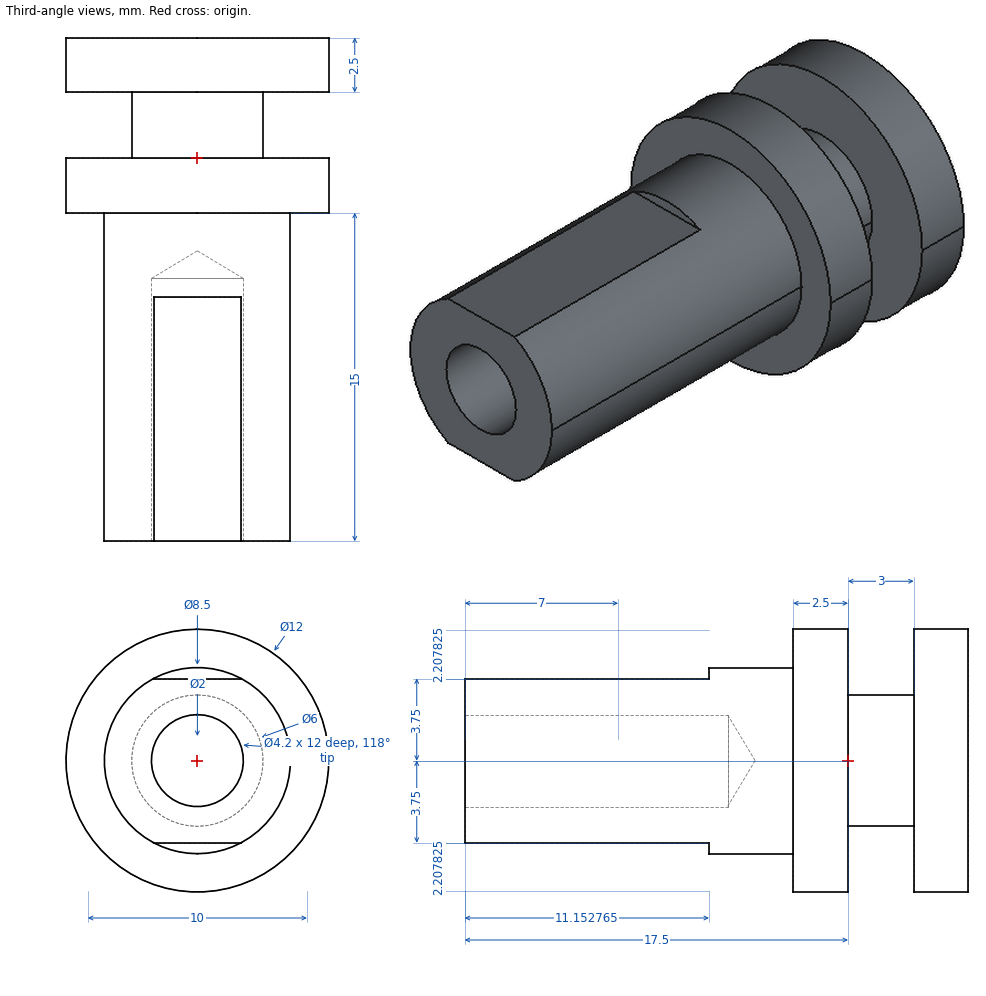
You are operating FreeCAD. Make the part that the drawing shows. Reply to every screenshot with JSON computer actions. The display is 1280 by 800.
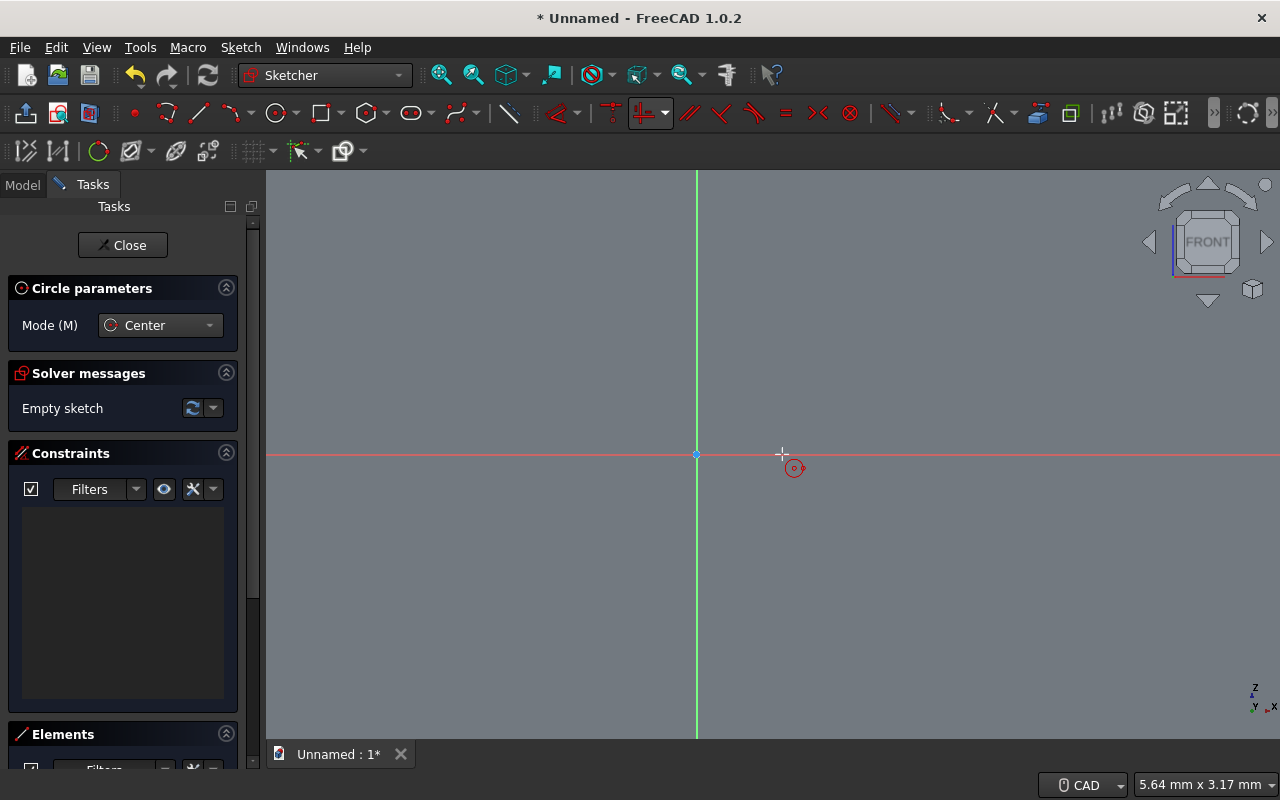
{"action": "left_click", "coordinate": [697, 454]}
{"action": "mouse_move", "coordinate": [824, 327]}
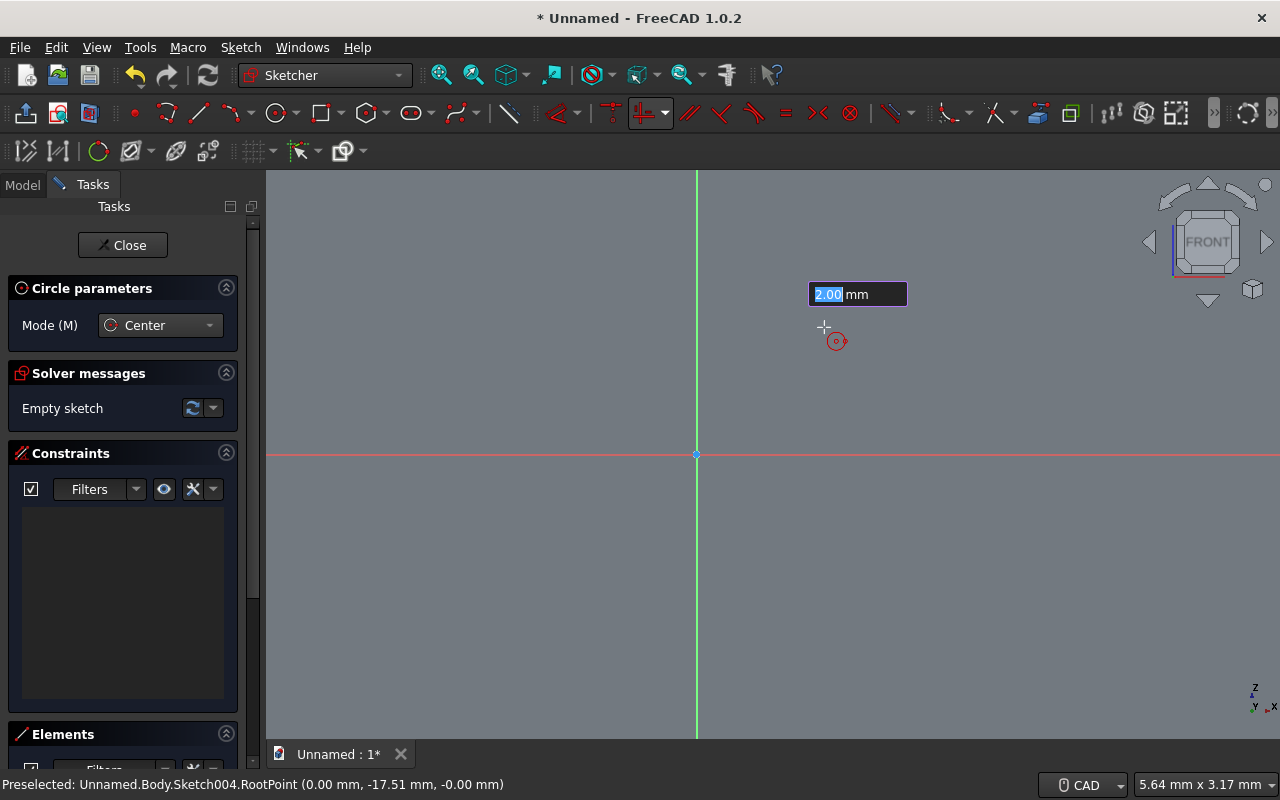
{"action": "type", "text": "2"}
{"action": "key", "text": "Return"}
{"action": "key", "text": "Escape"}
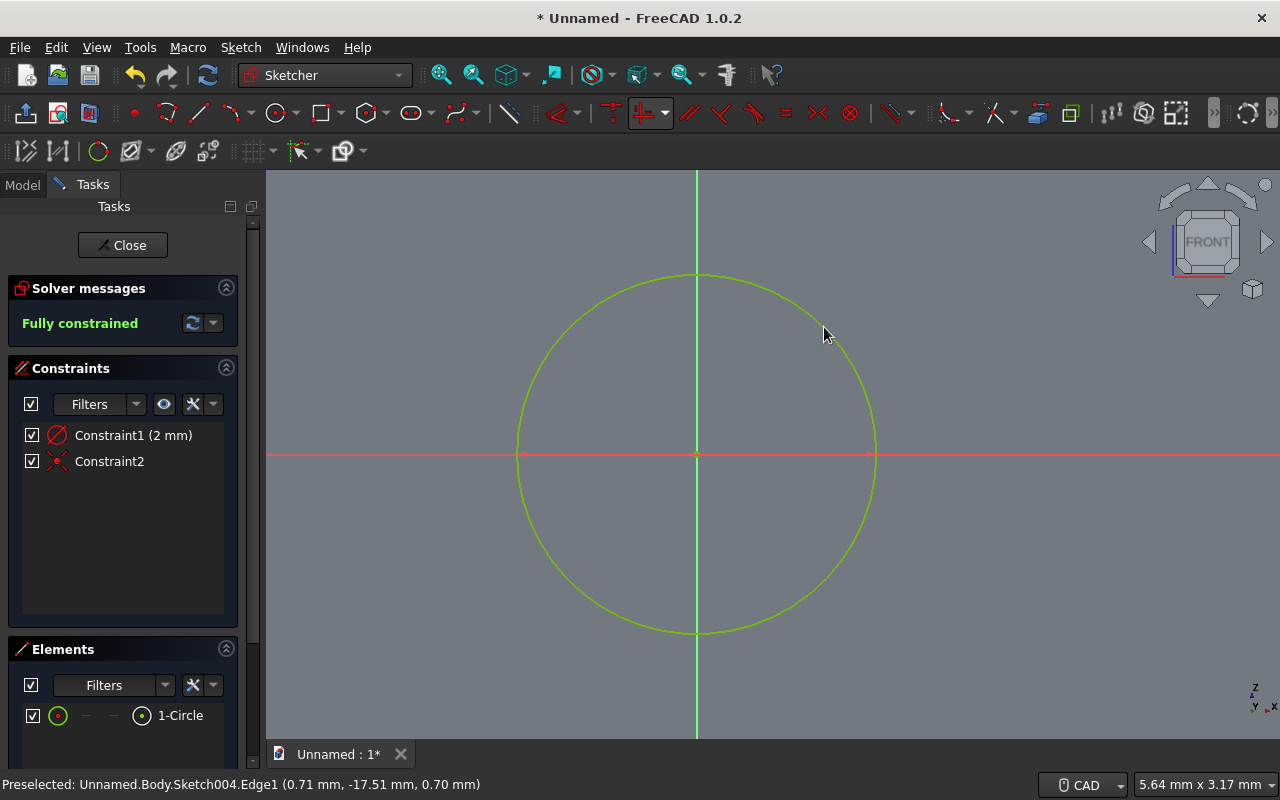
{"action": "left_click", "coordinate": [123, 245]}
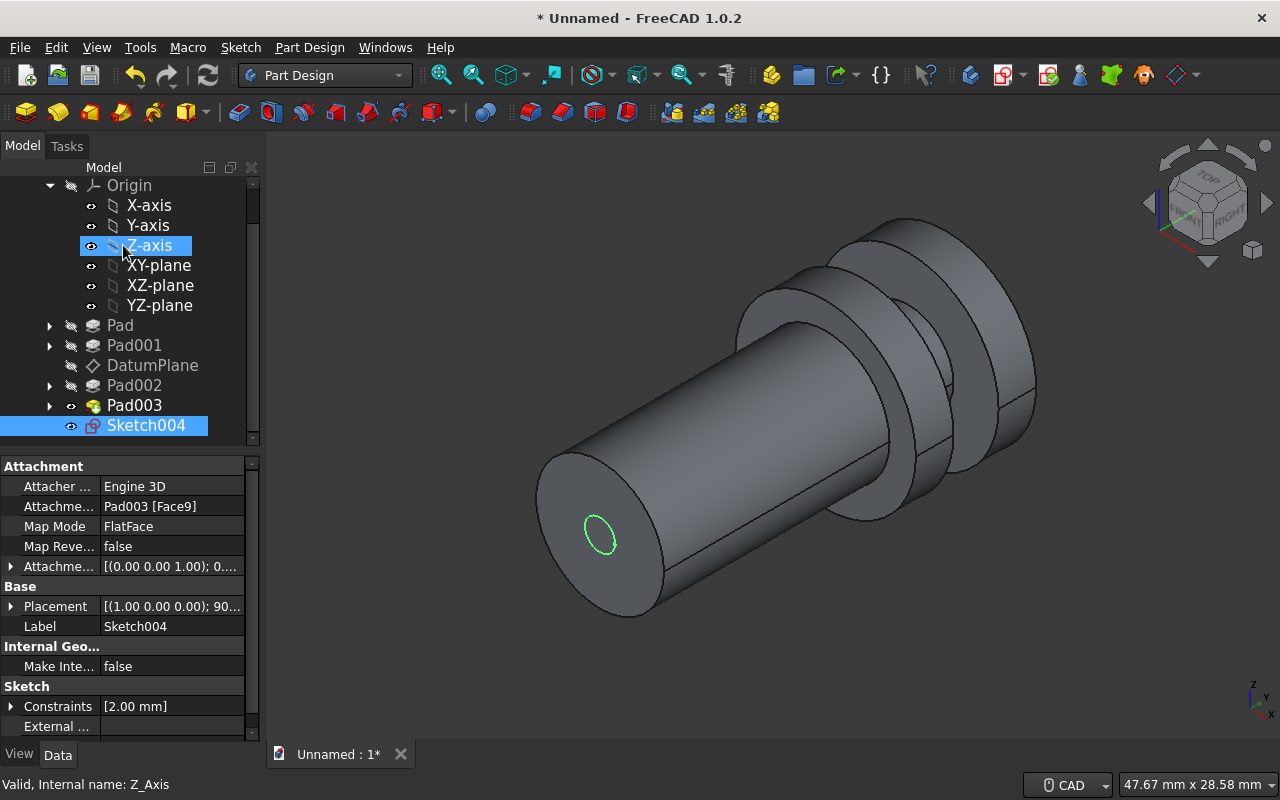
{"action": "left_click", "coordinate": [240, 112]}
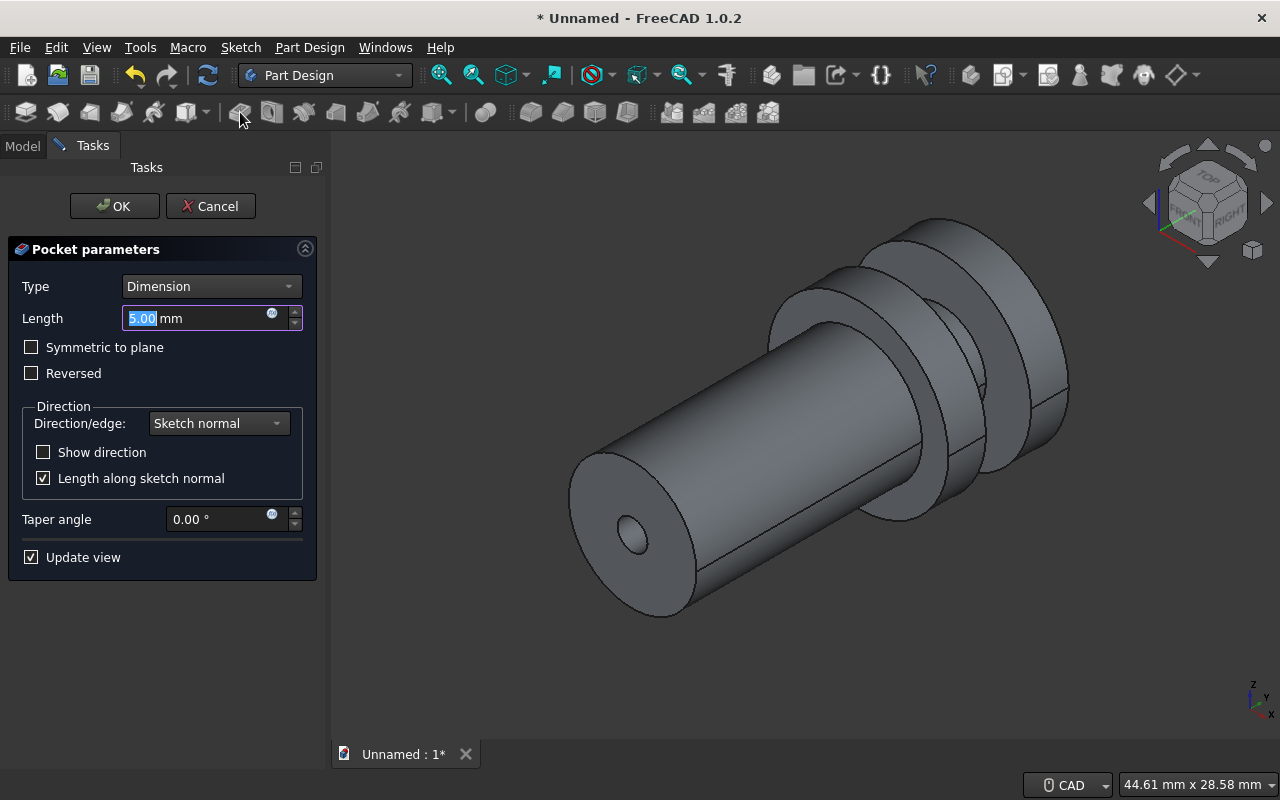
{"action": "type", "text": "7"}
{"action": "key", "text": "Tab"}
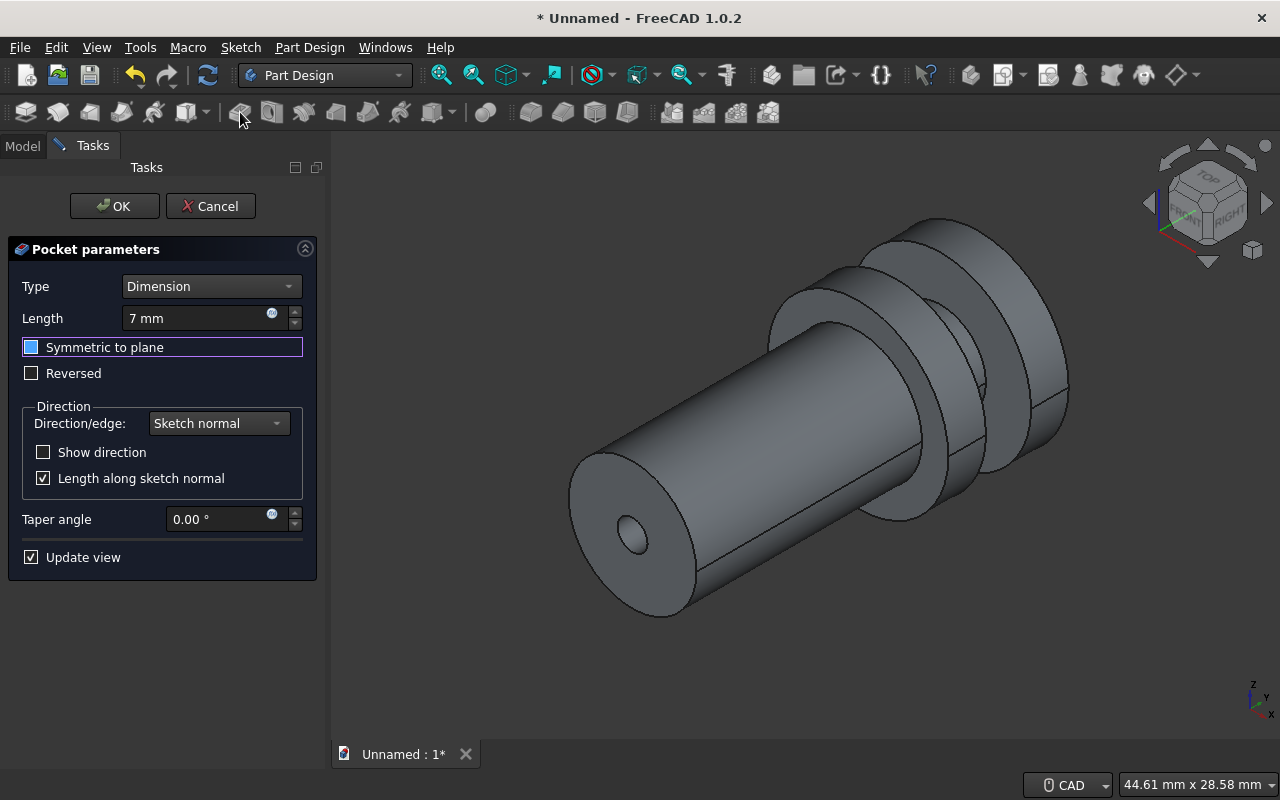
{"action": "left_click", "coordinate": [115, 206]}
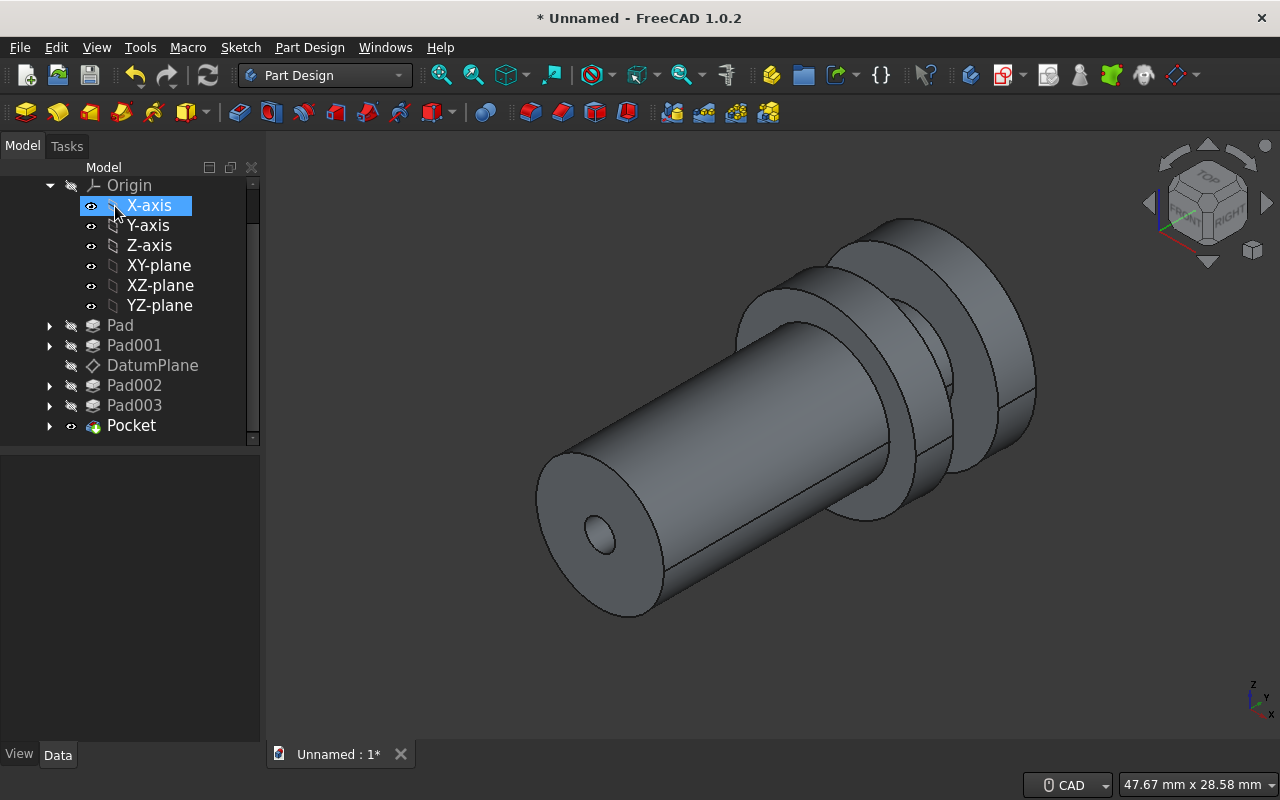
{"action": "left_click", "coordinate": [618, 587]}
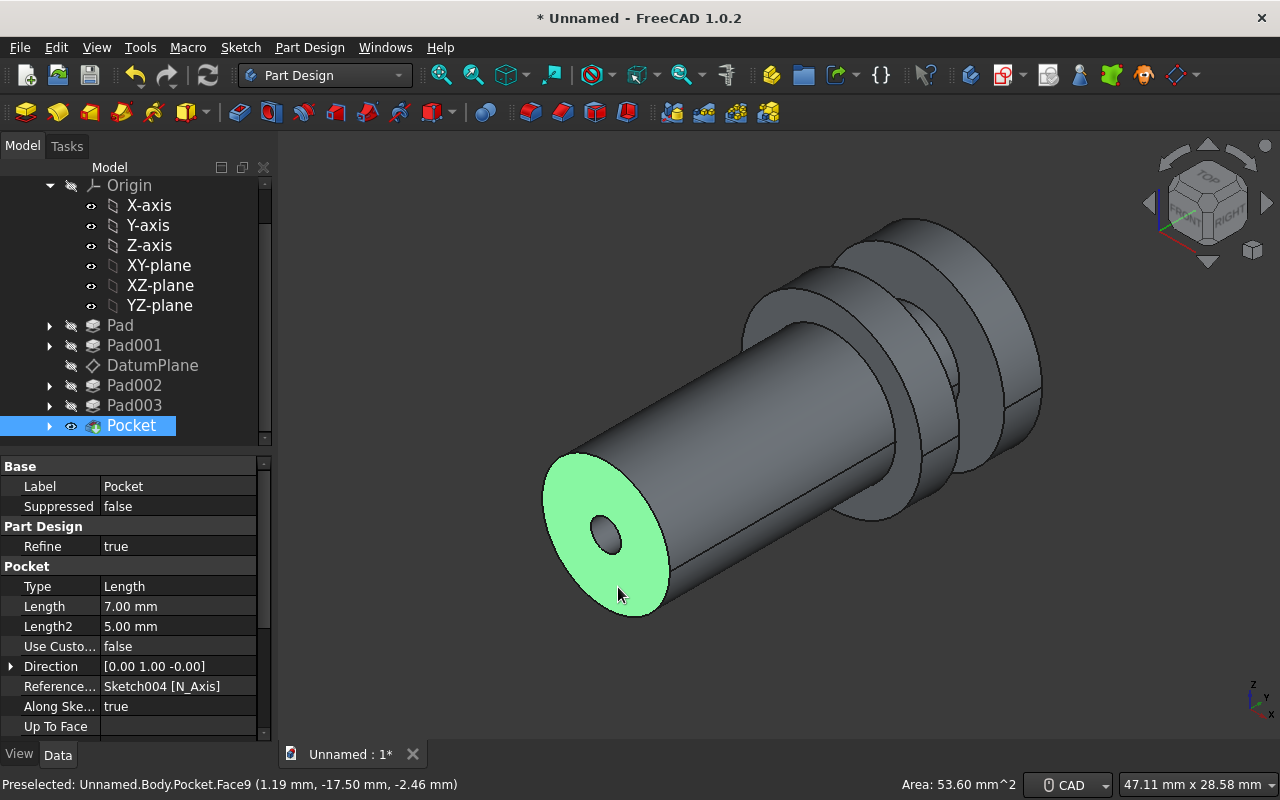
{"action": "left_click", "coordinate": [1004, 76]}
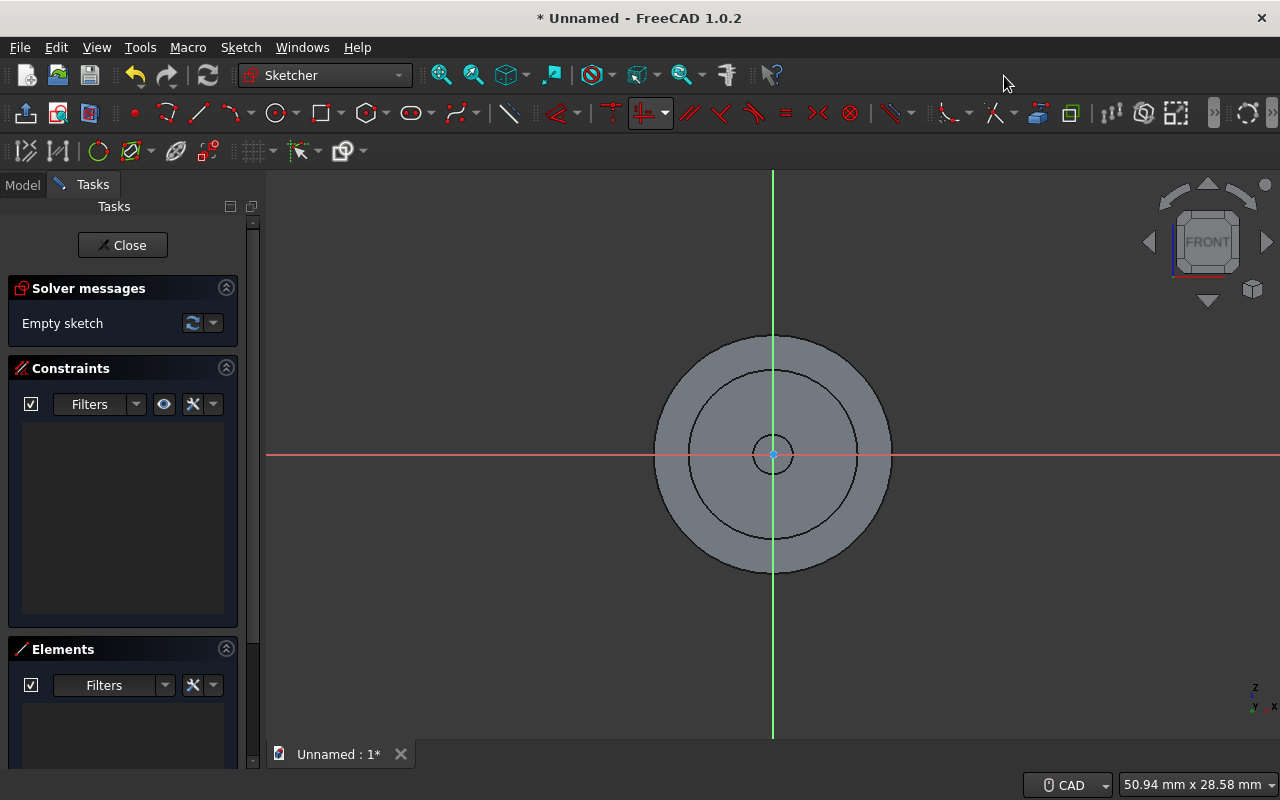
{"action": "scroll", "coordinate": [795, 454], "scroll_direction": "up", "scroll_amount": 7}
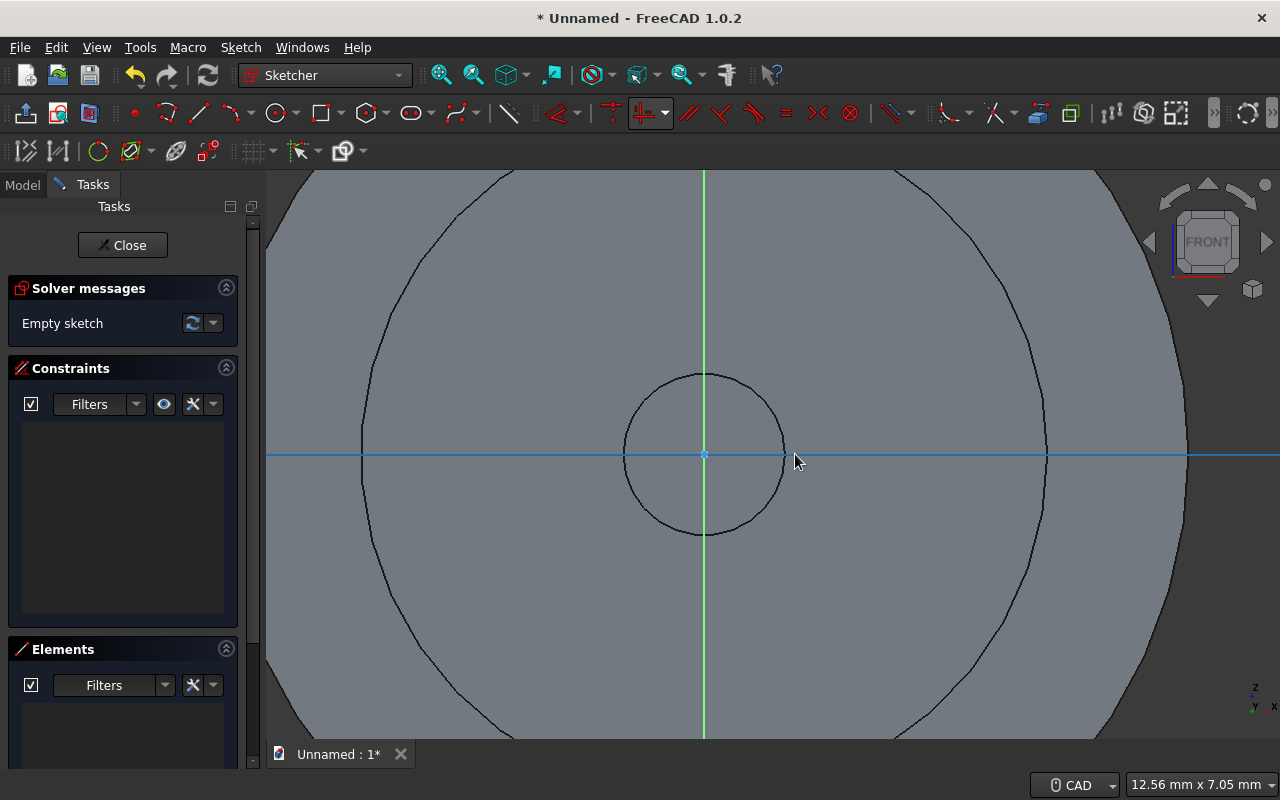
{"action": "key", "text": "g c"}